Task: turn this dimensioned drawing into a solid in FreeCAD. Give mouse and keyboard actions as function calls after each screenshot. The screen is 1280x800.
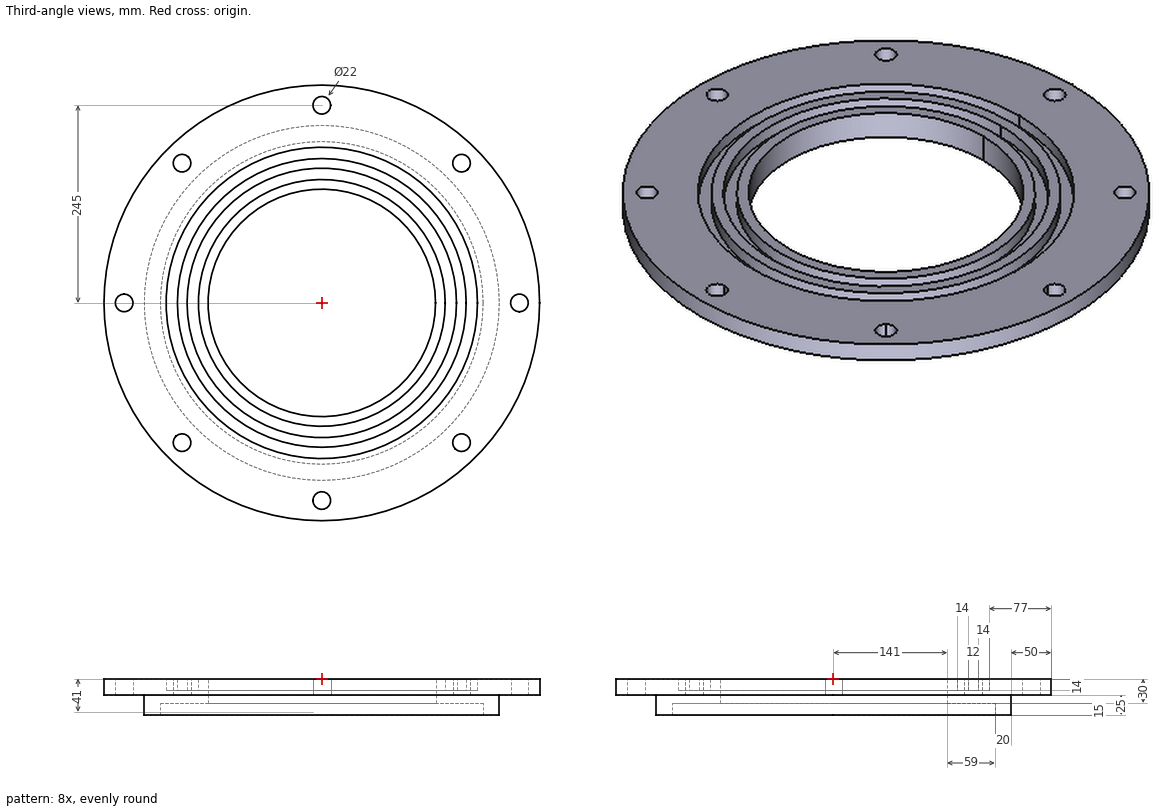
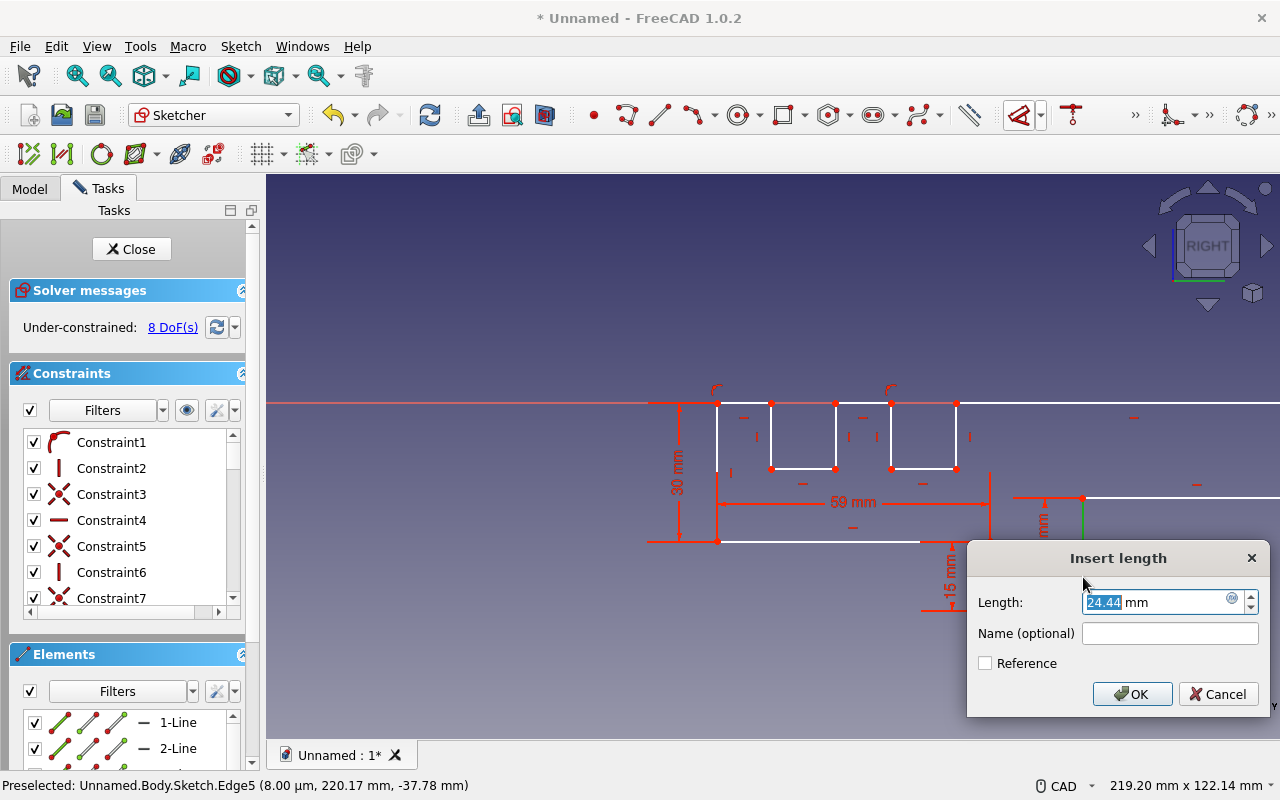
text(25)
key(Return)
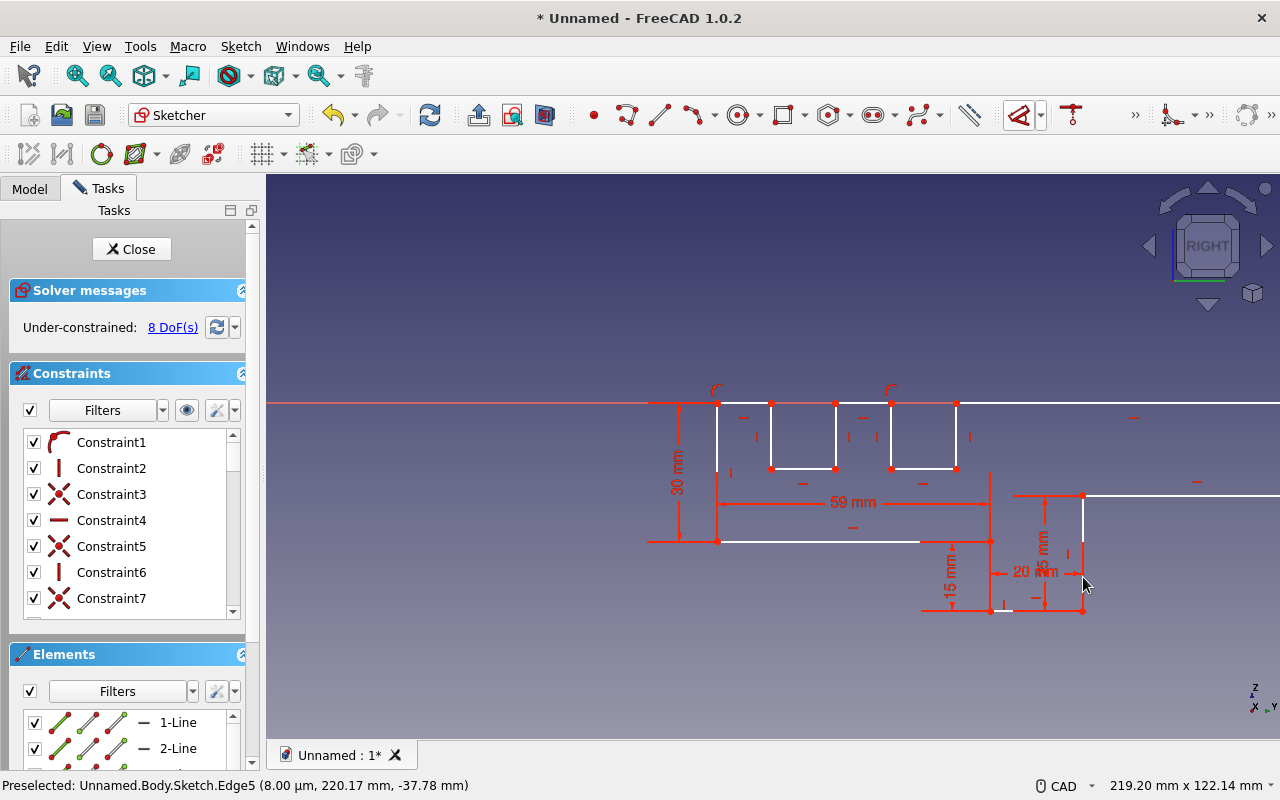
scroll(717, 415, down, 4)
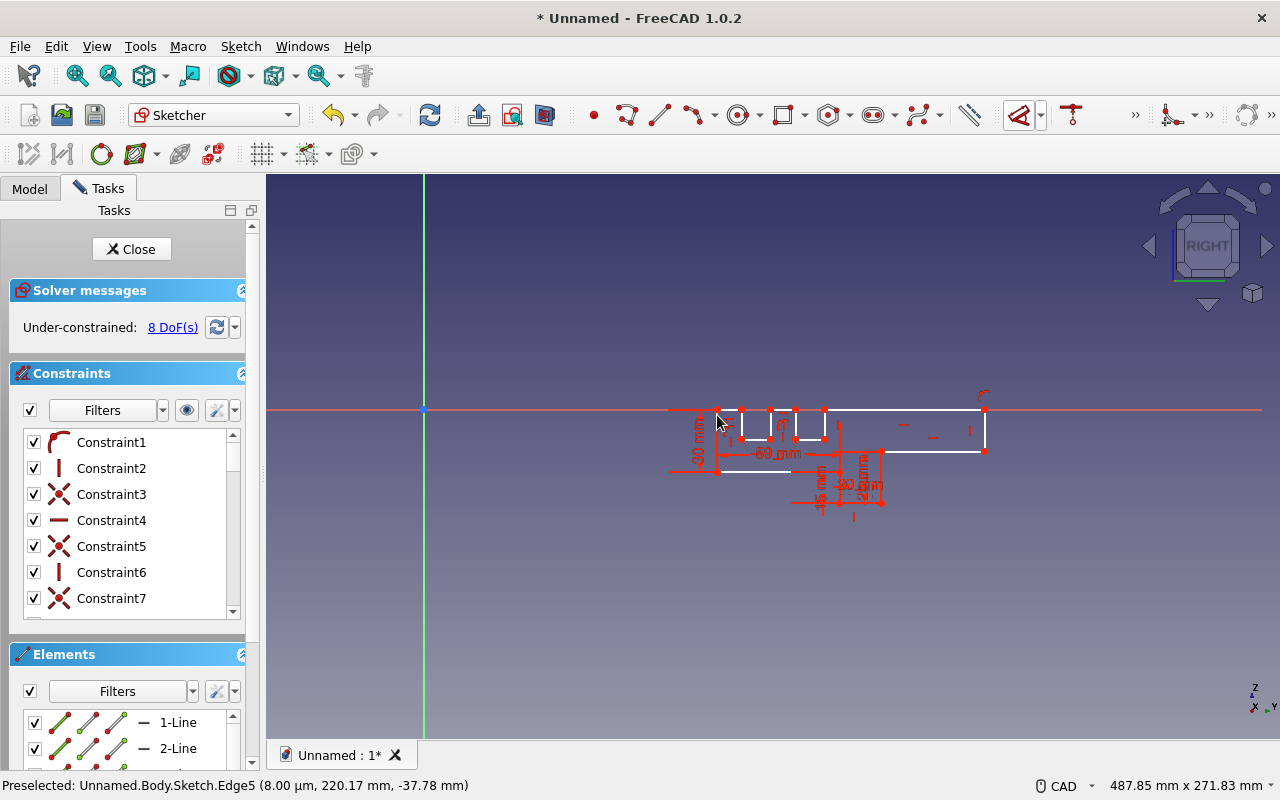
click(912, 452)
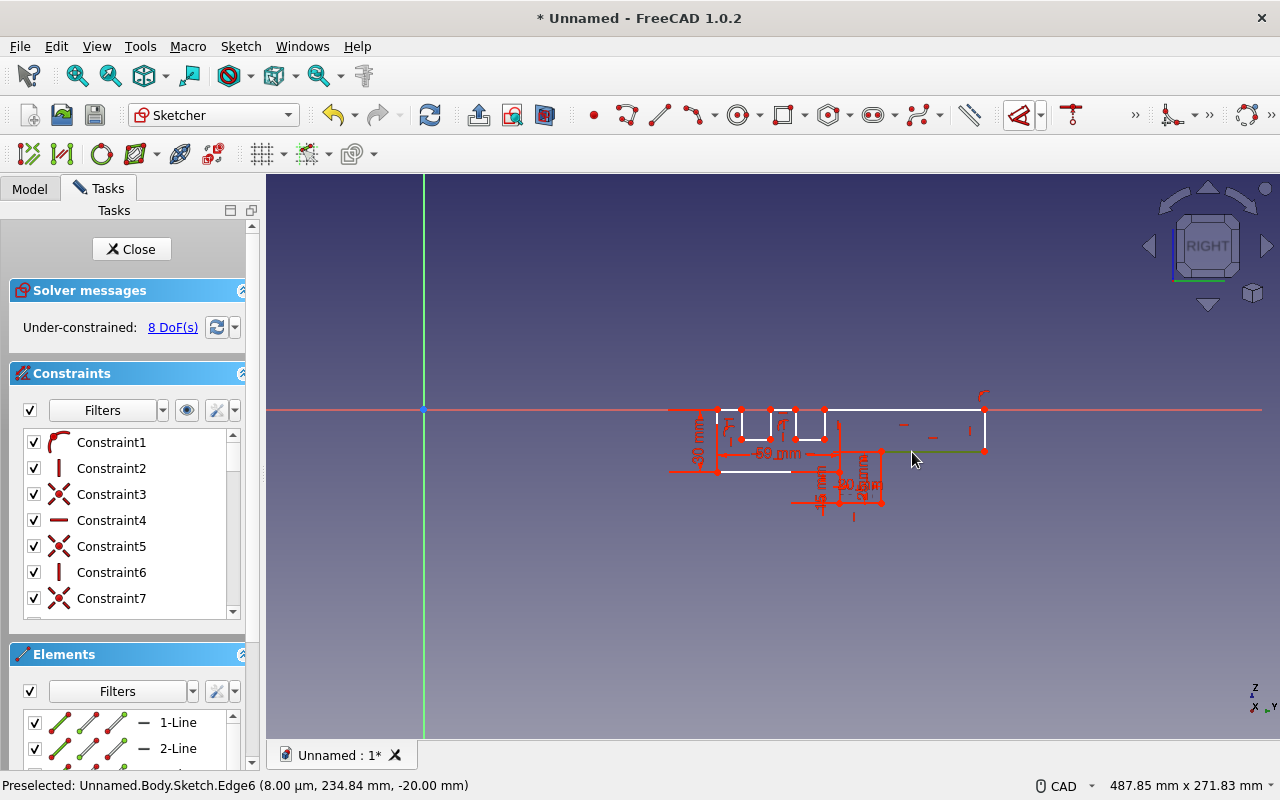
key(l)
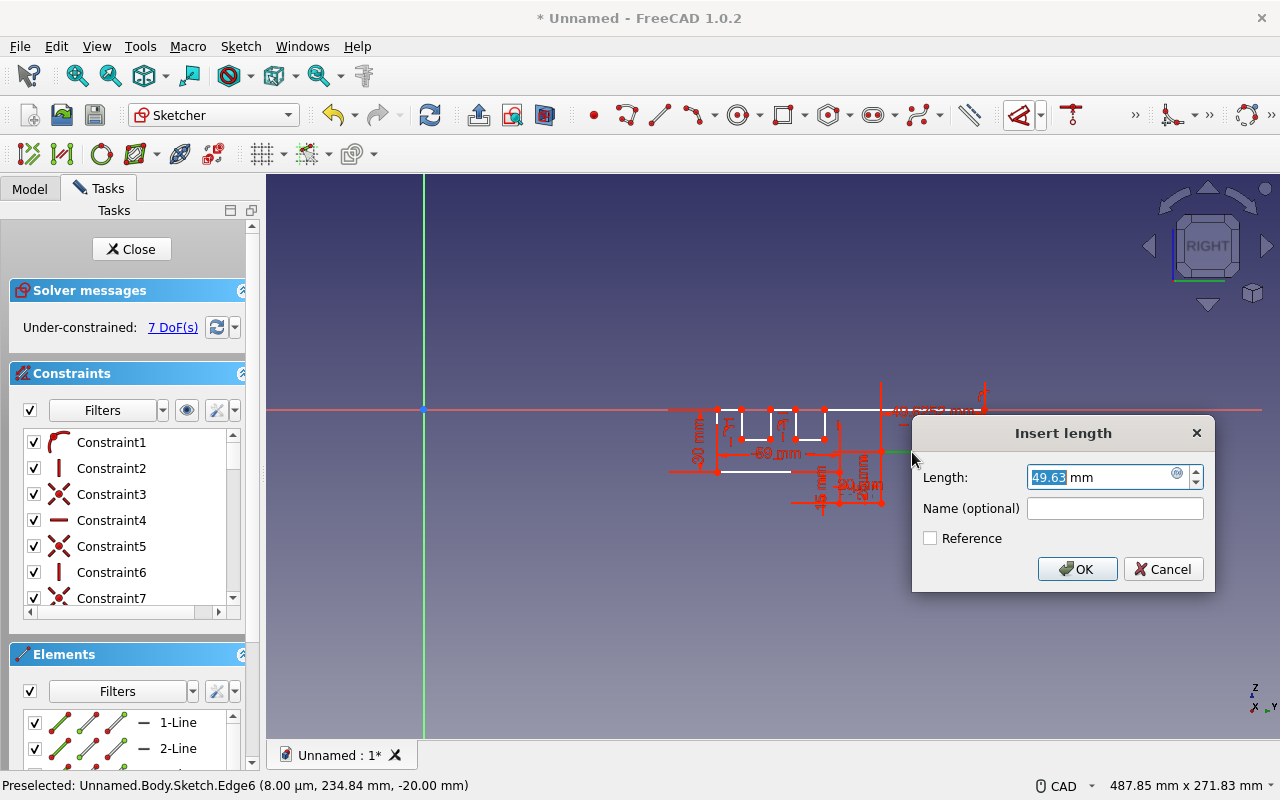
text(50)
key(Return)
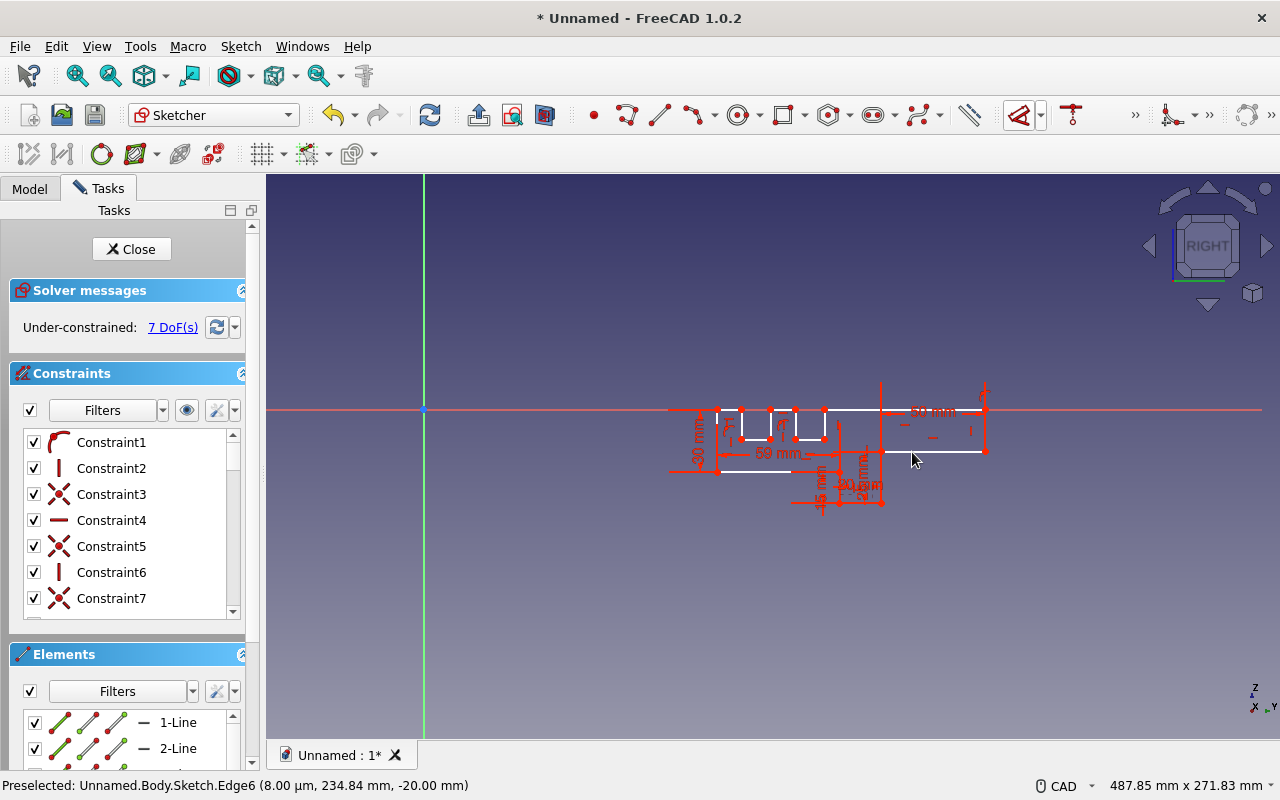
click(873, 410)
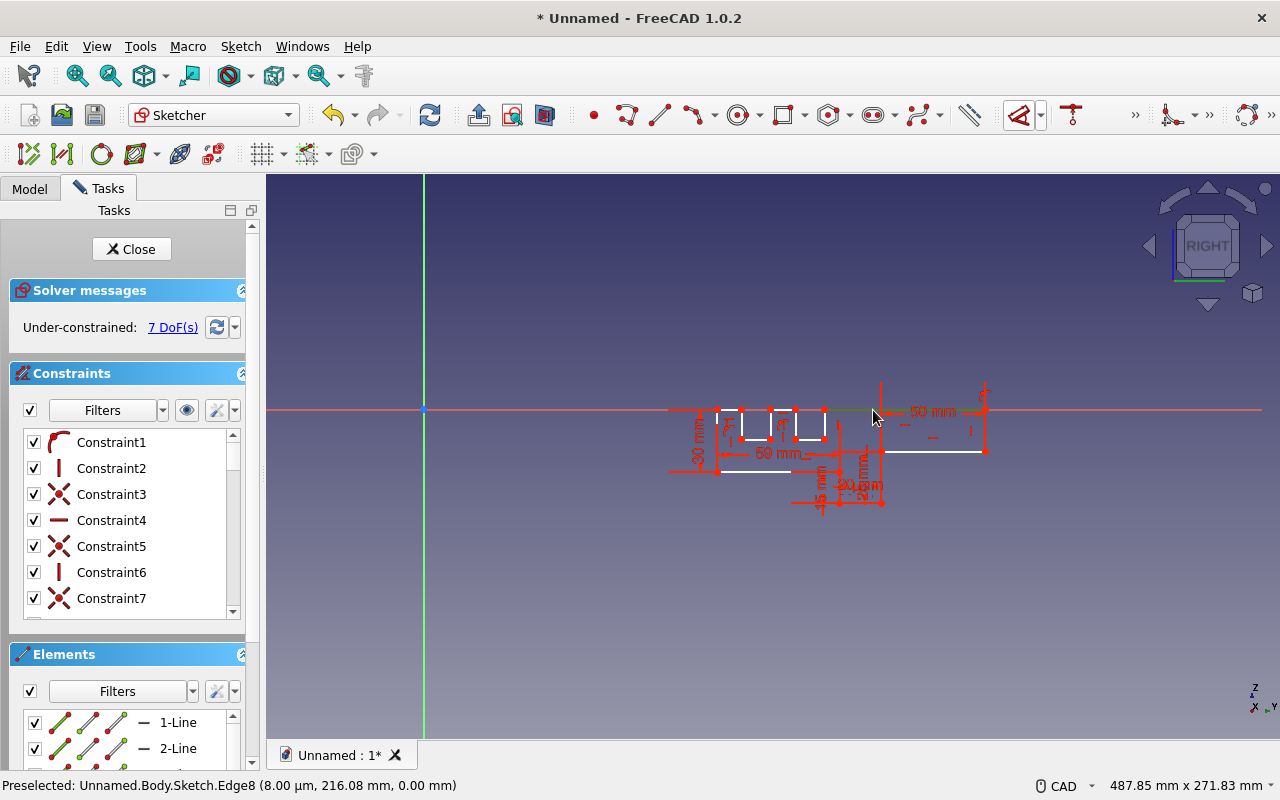
click(1040, 116)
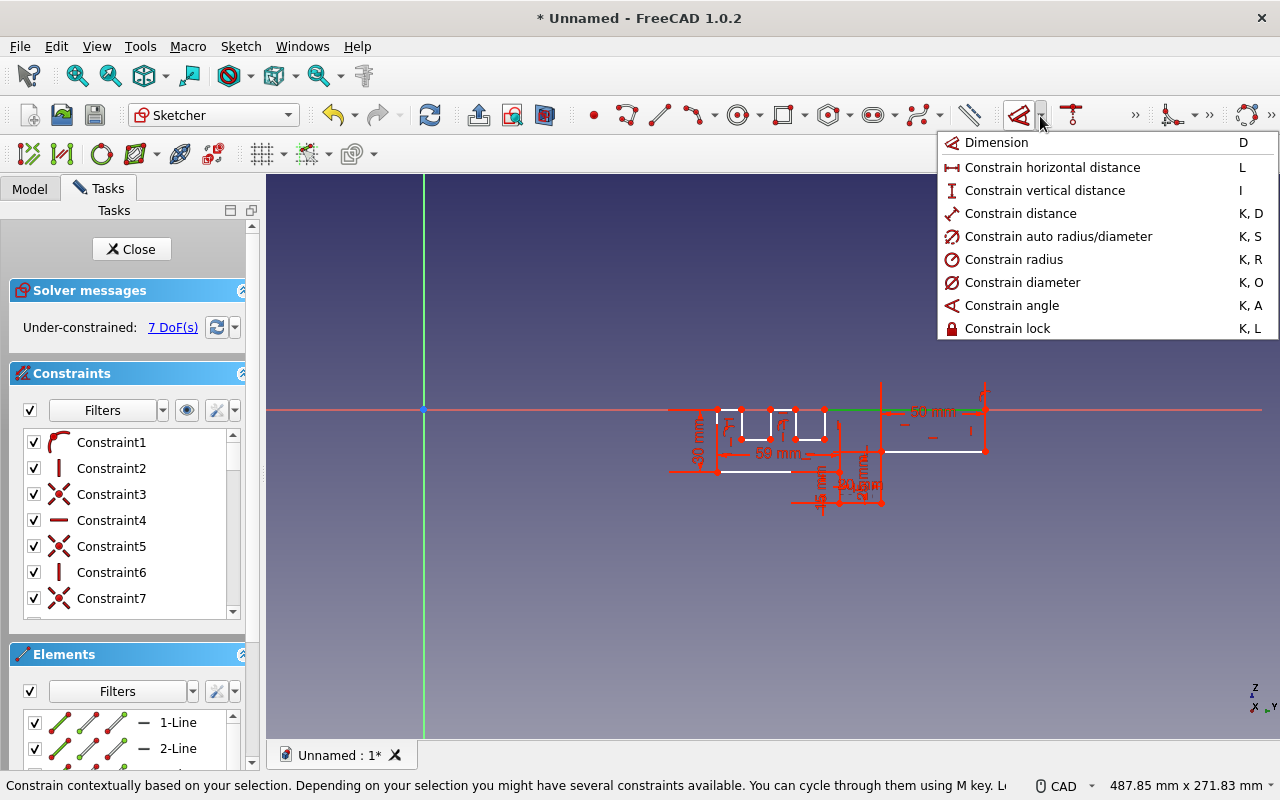
click(1108, 168)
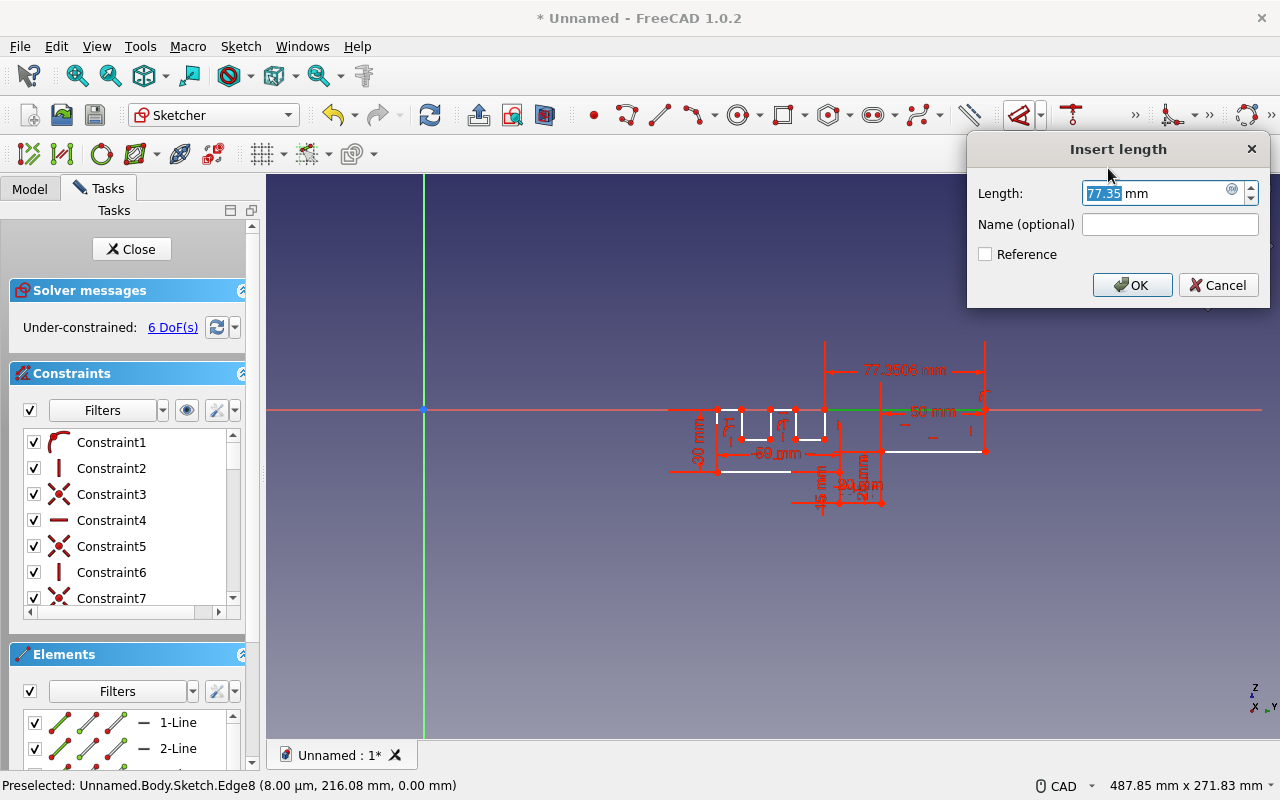
text(77)
key(Return)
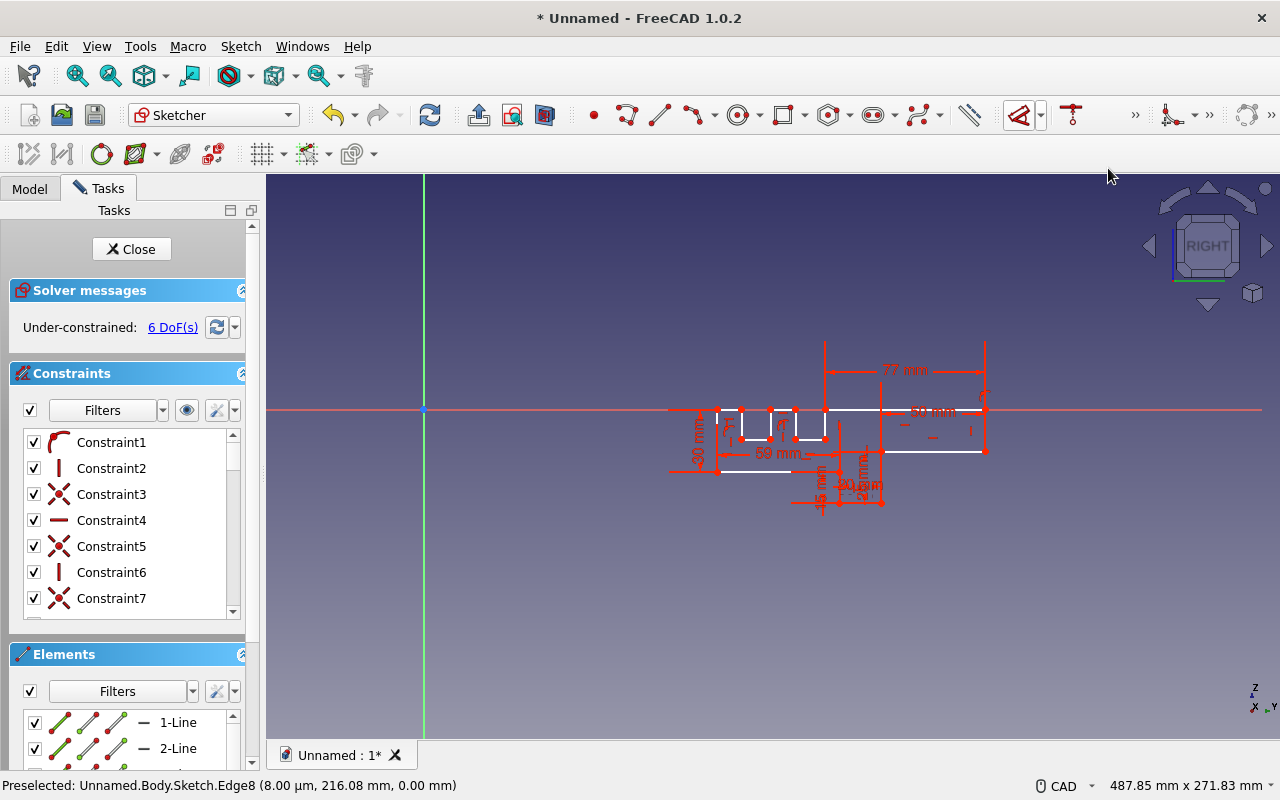
scroll(825, 422, up, 2)